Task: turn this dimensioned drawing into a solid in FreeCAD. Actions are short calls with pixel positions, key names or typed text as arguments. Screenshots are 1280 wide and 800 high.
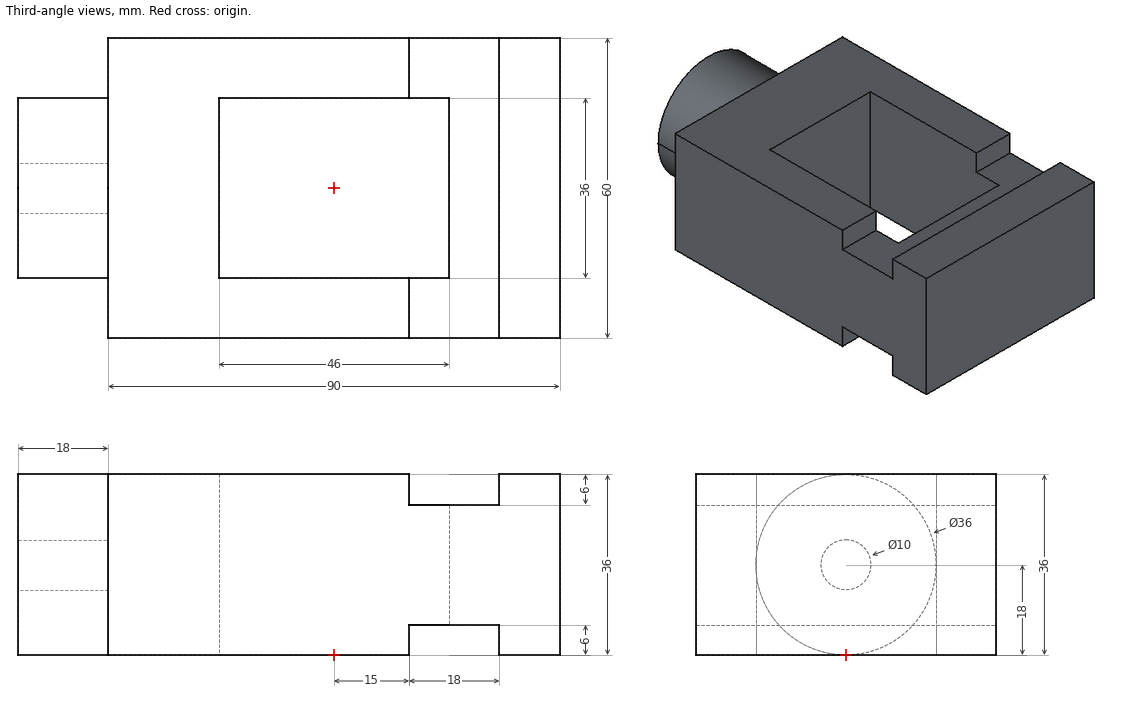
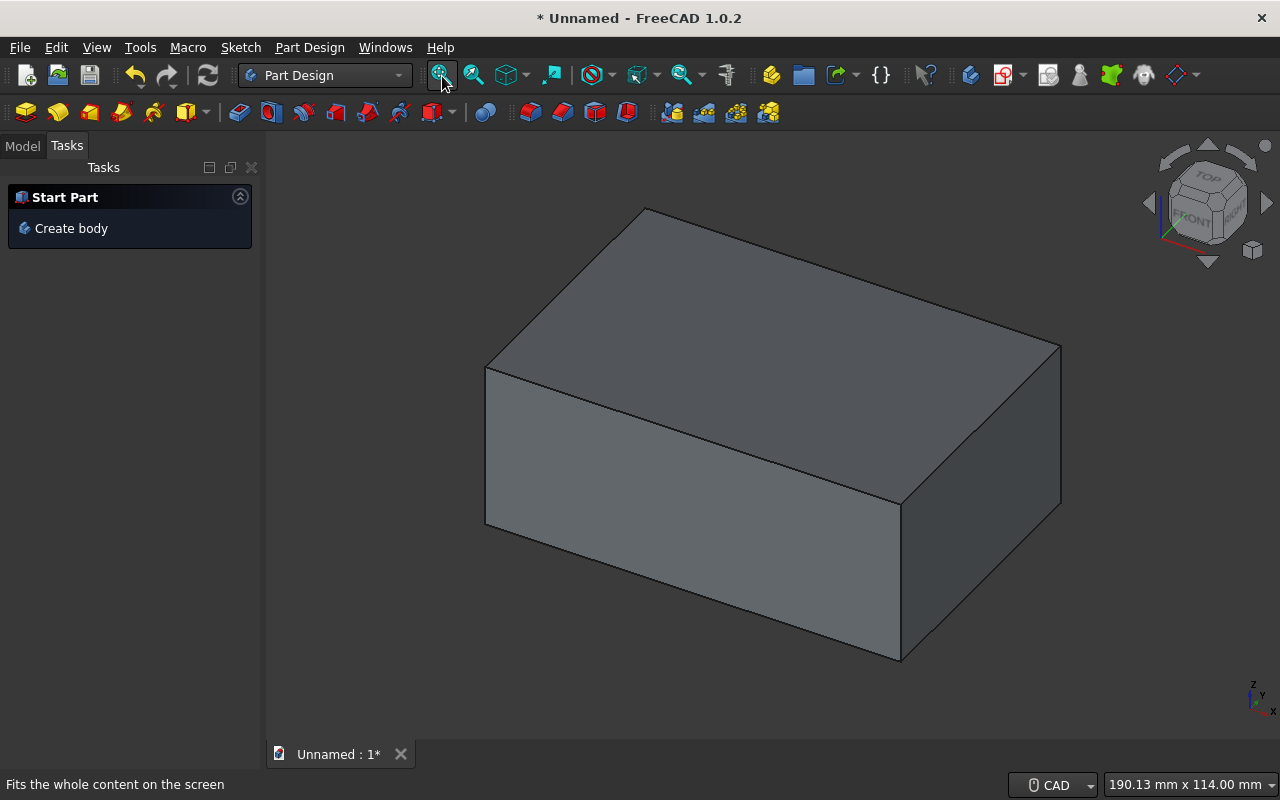
click(832, 375)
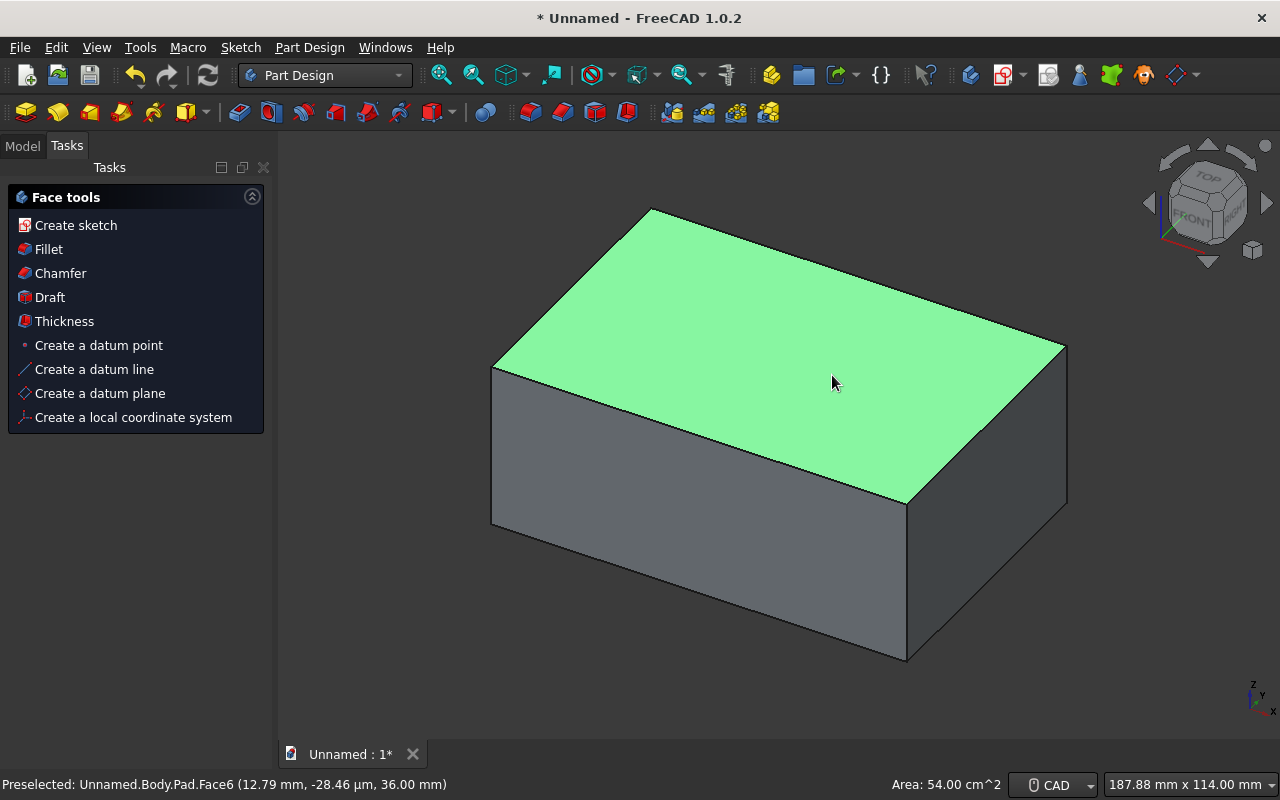
click(1004, 76)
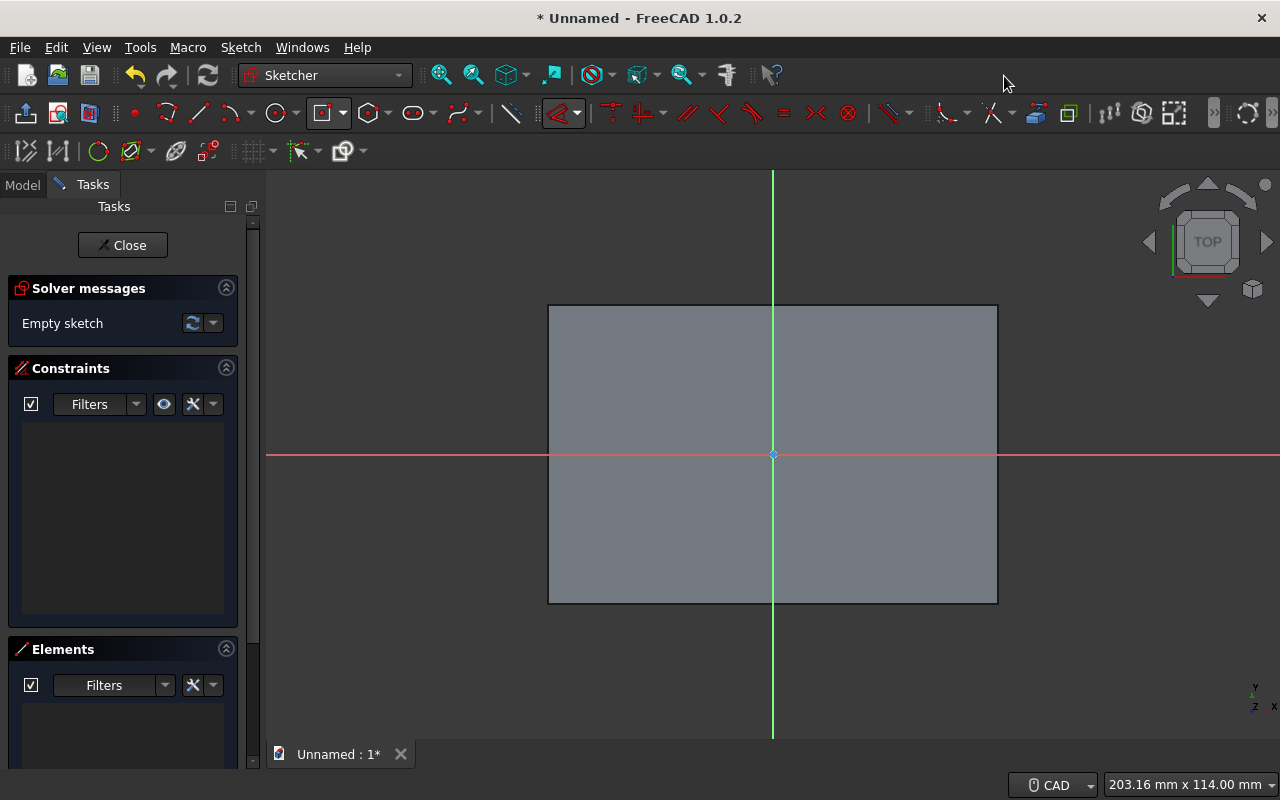
scroll(829, 455, up, 4)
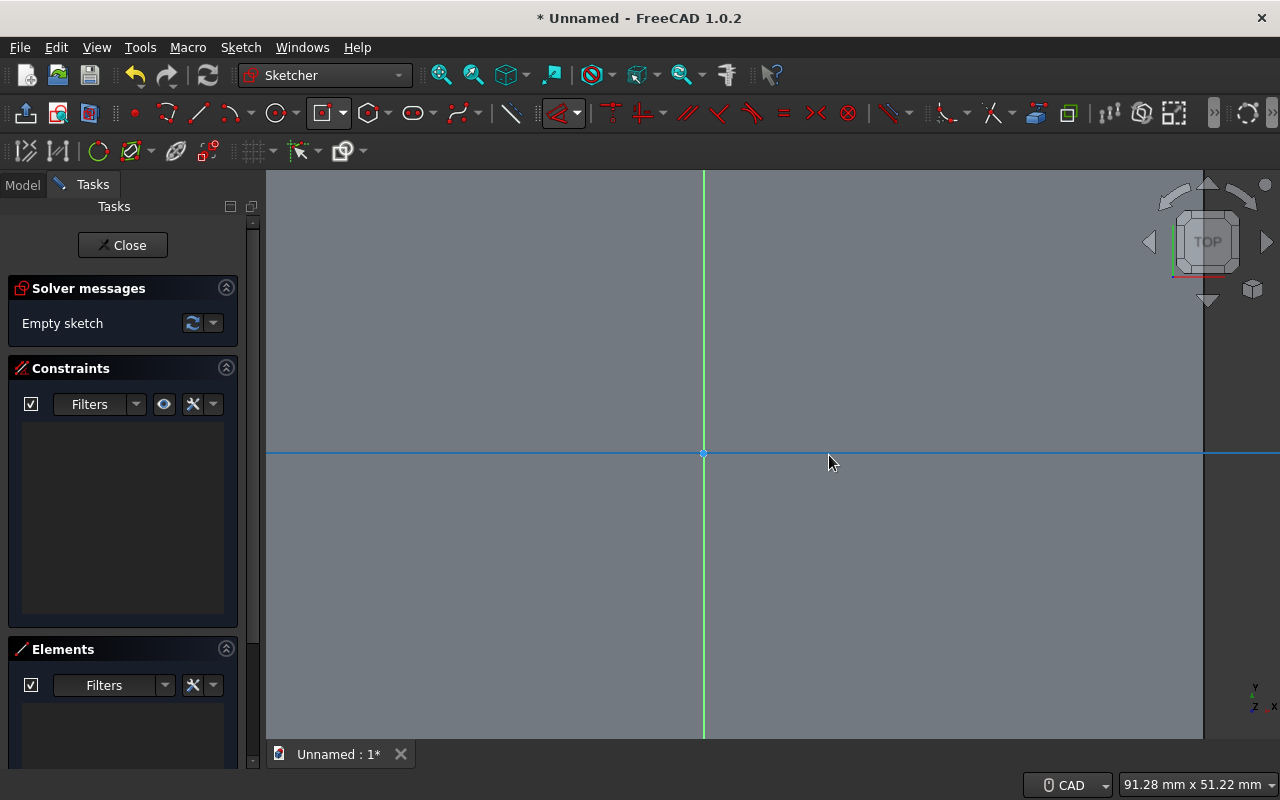
click(322, 114)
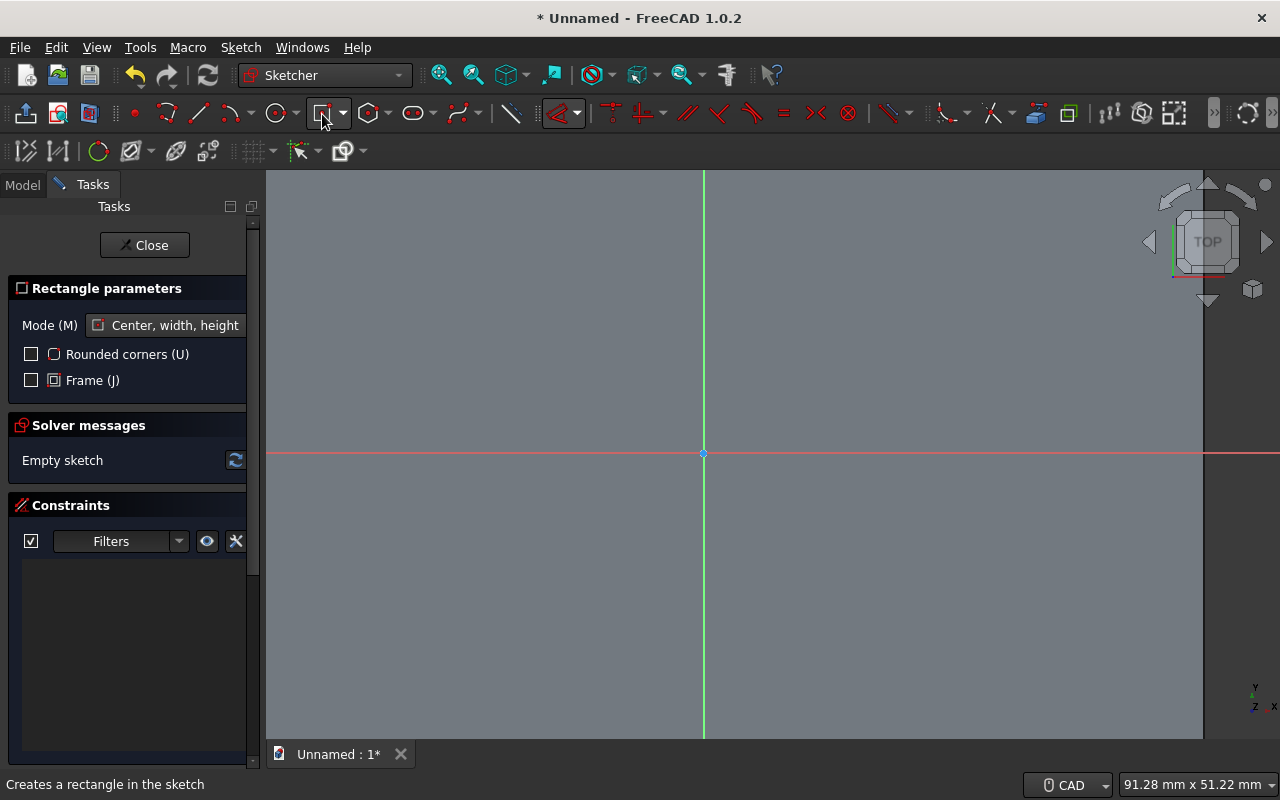
click(704, 453)
click(959, 253)
key(Escape)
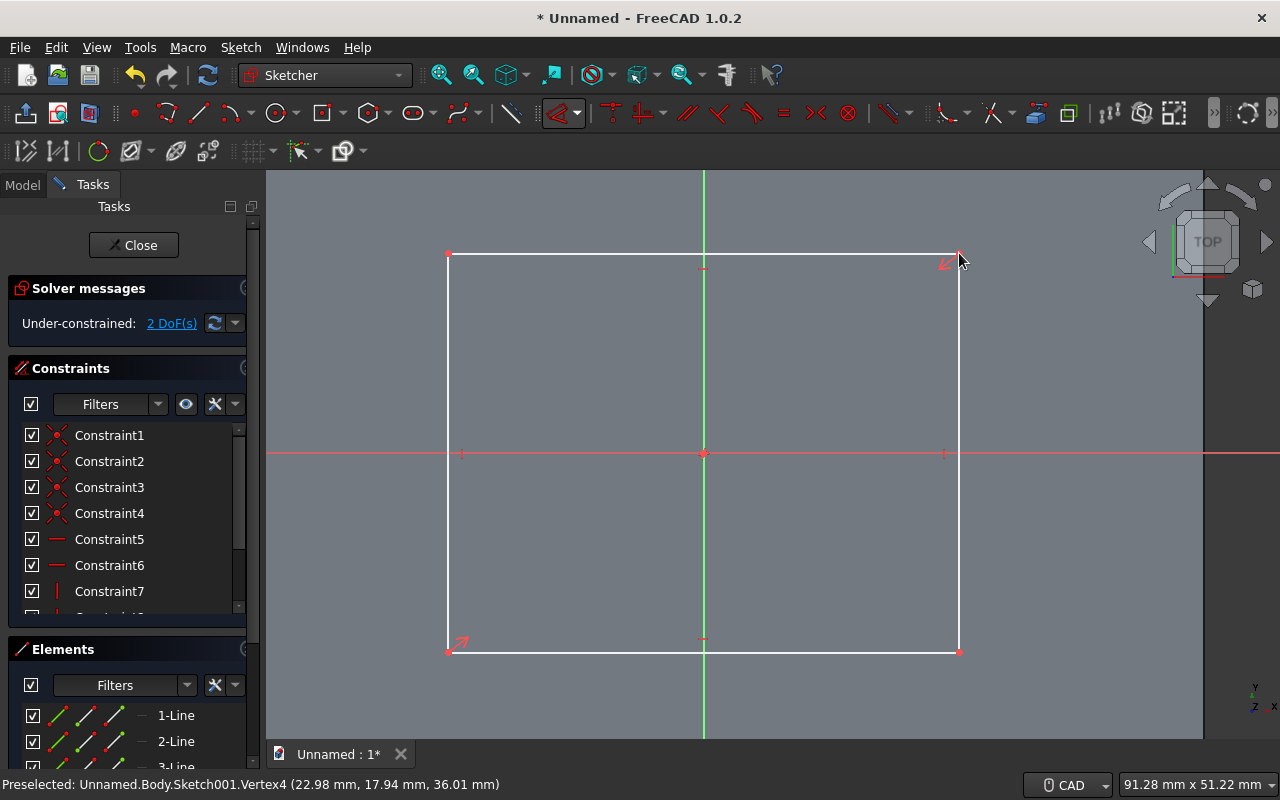
click(602, 653)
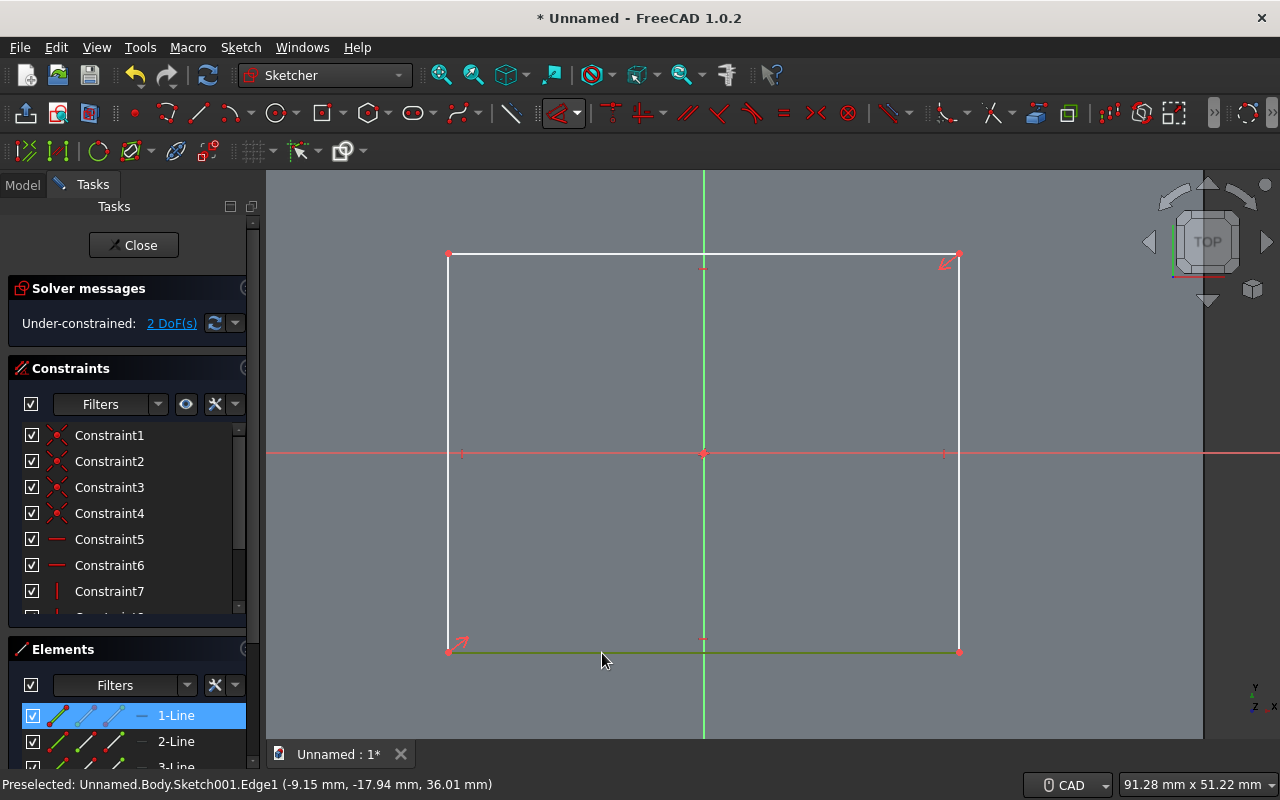
key(l)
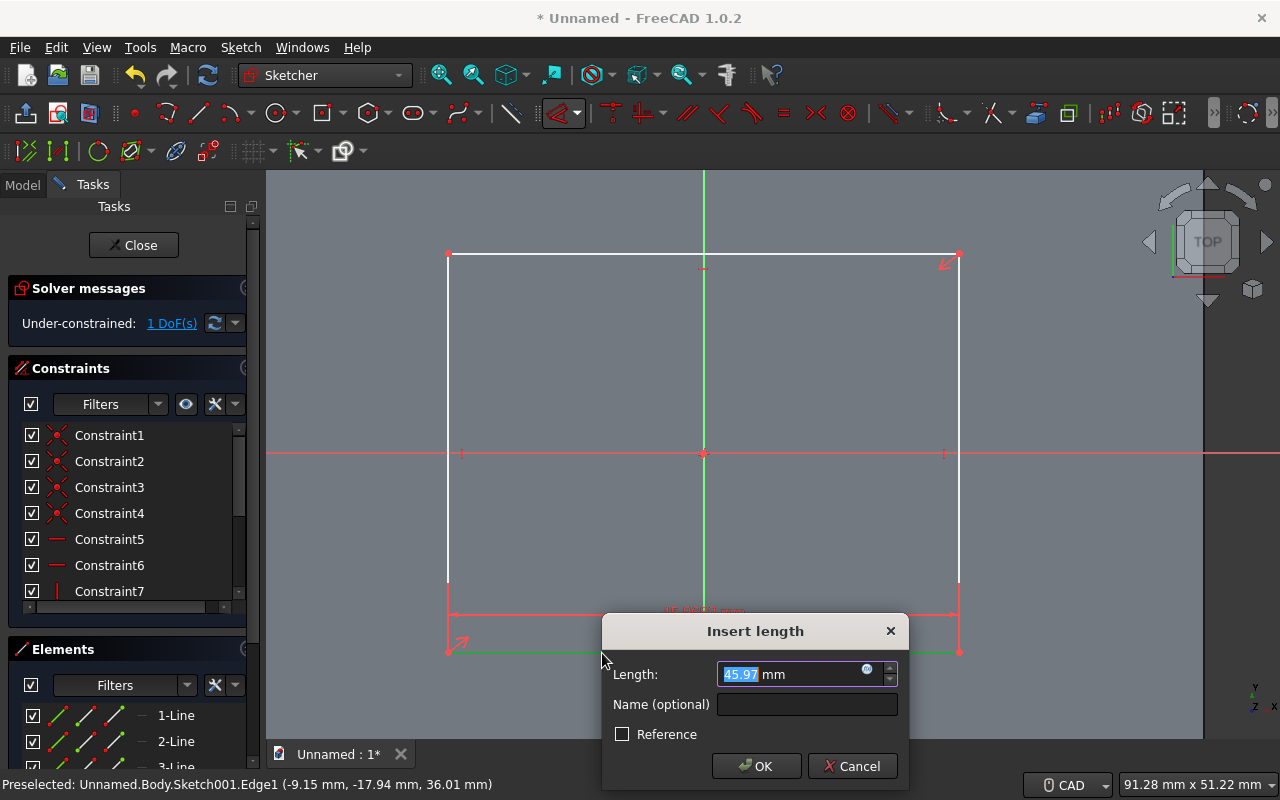
text(46)
key(Return)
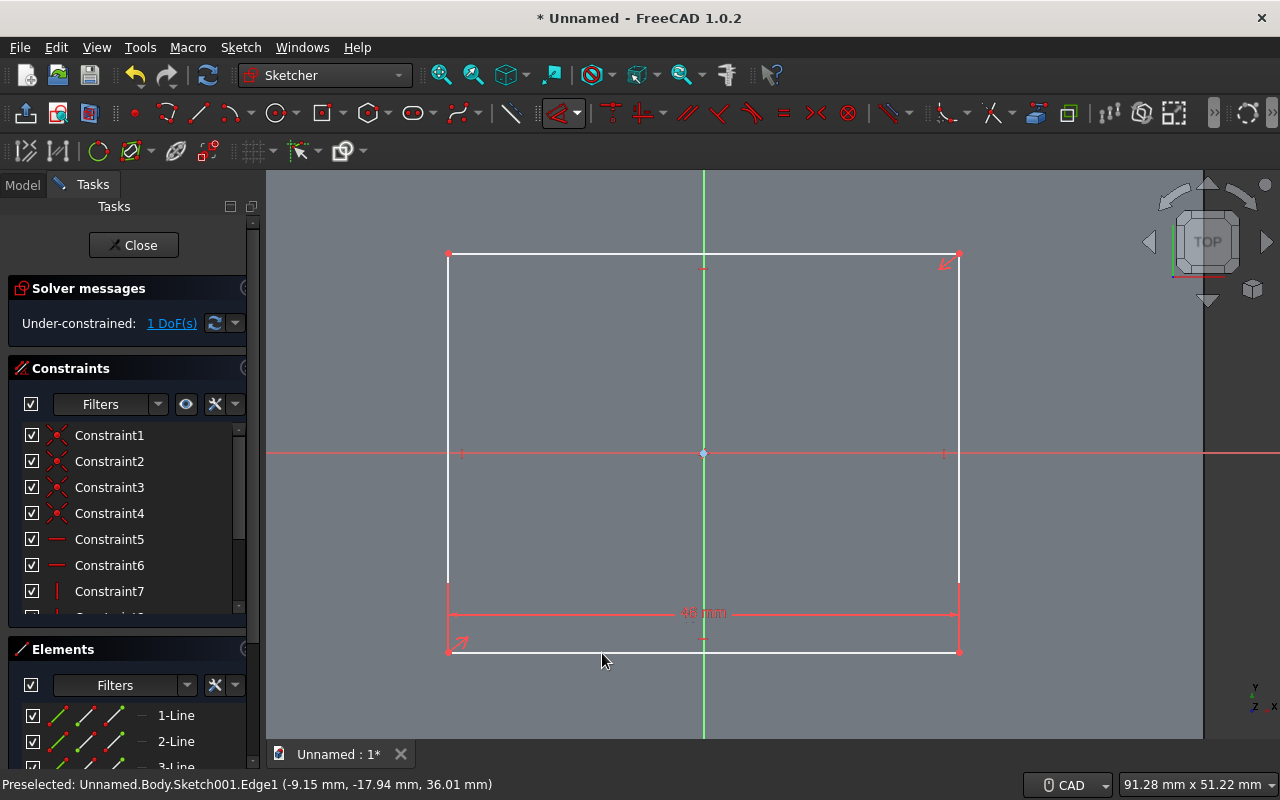
click(959, 533)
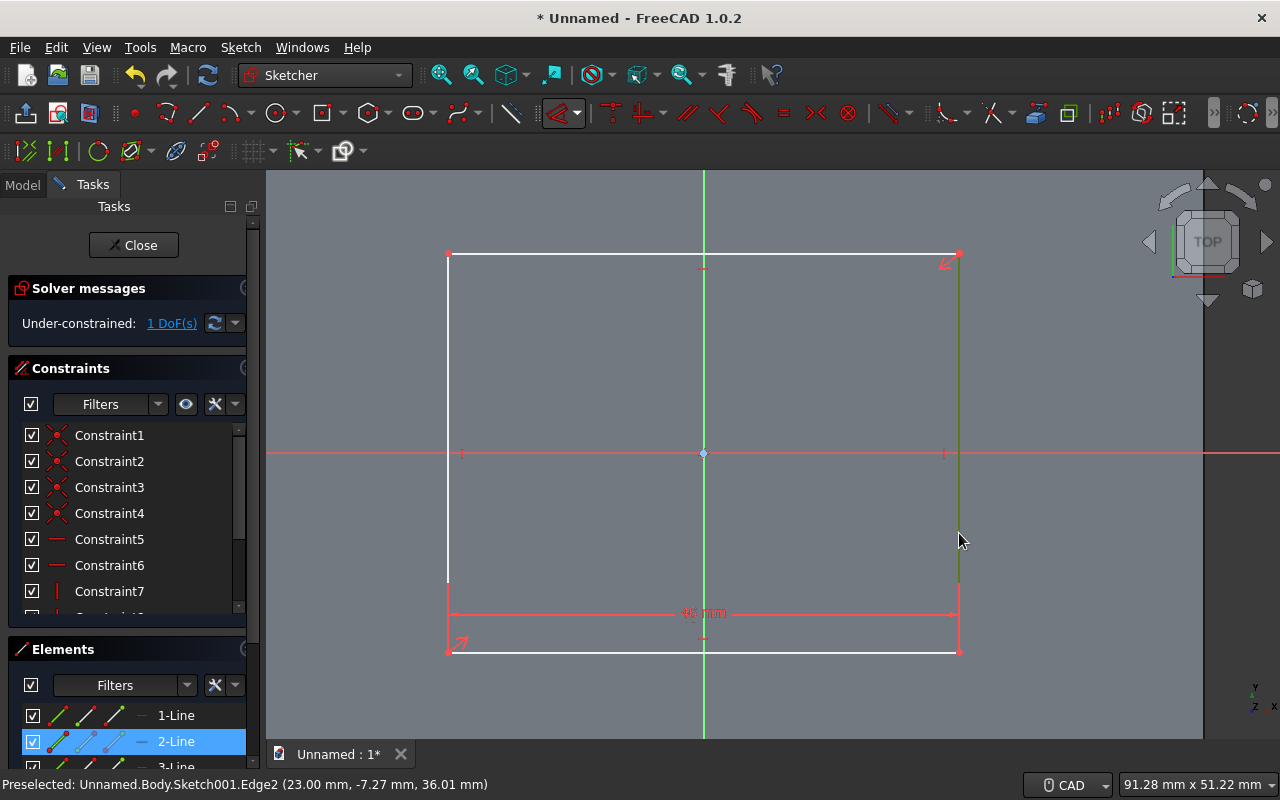
click(580, 114)